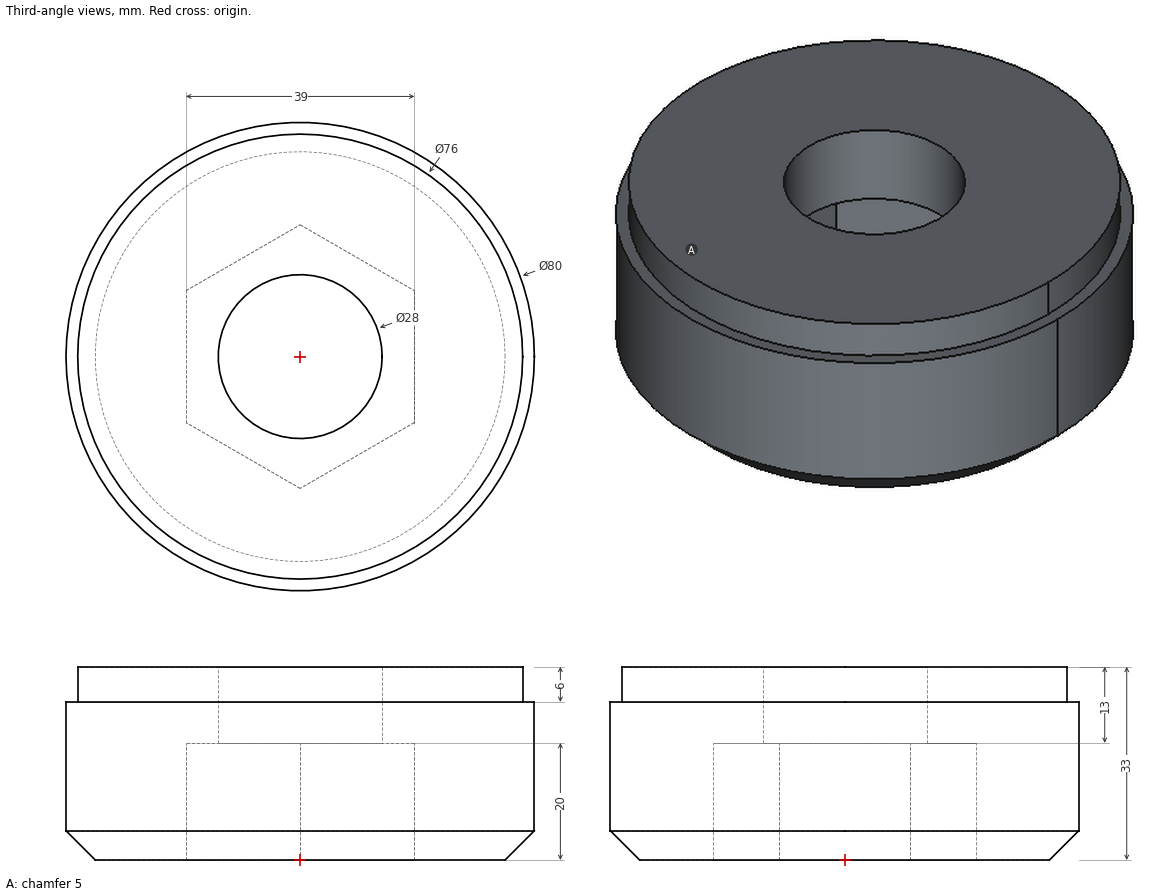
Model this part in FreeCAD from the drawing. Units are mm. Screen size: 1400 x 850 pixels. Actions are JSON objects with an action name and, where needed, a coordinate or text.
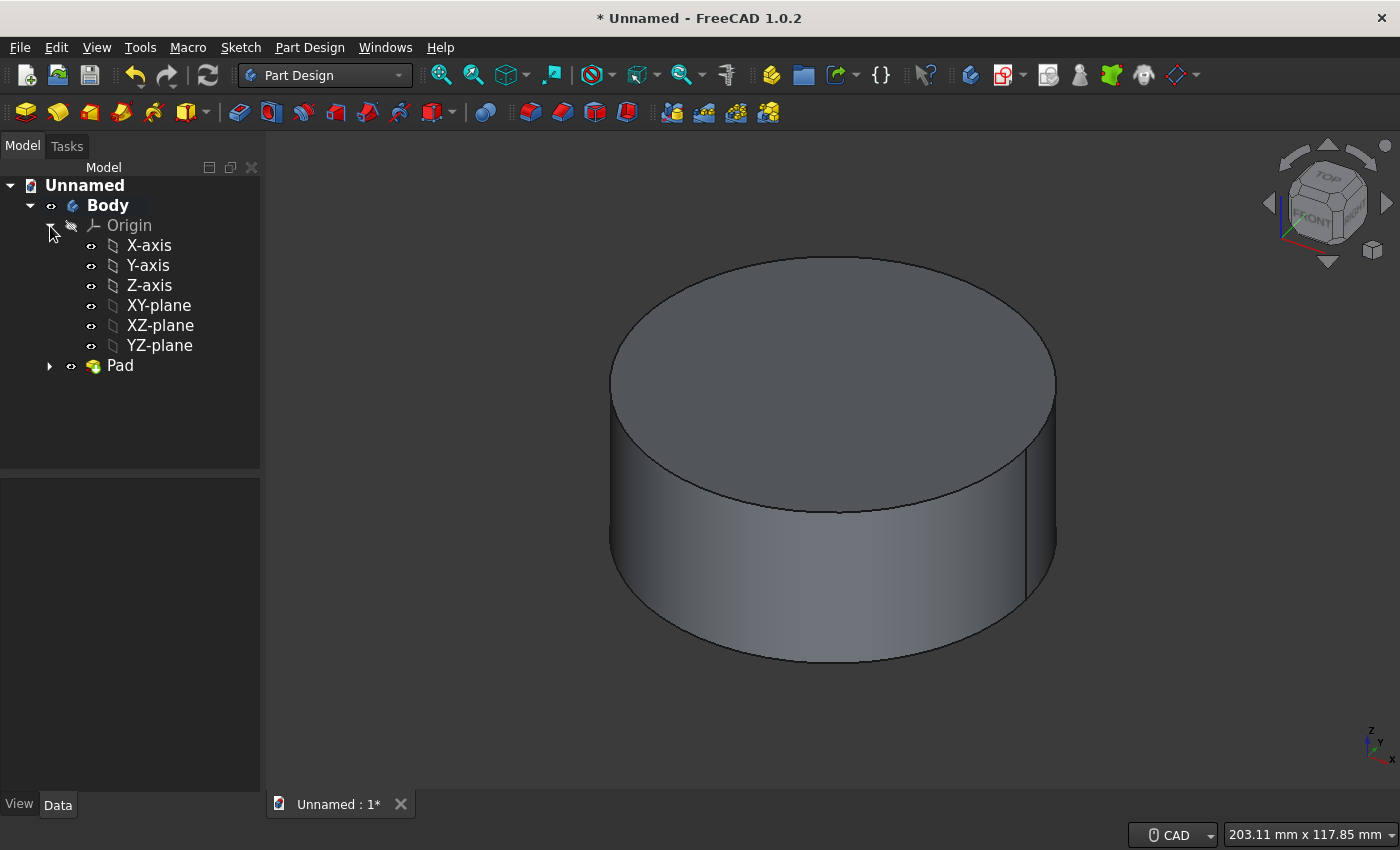
{"action": "left_click", "coordinate": [136, 306]}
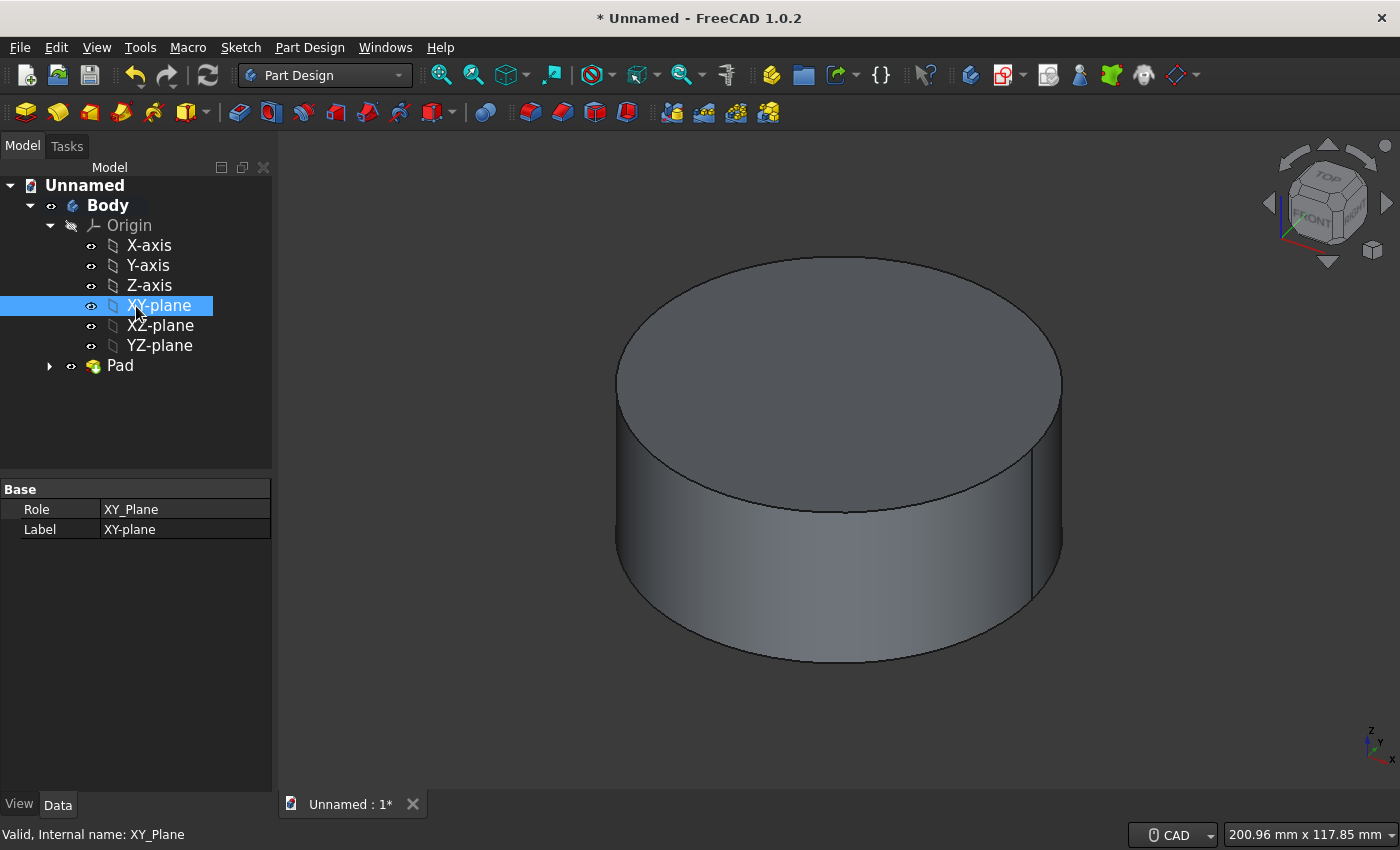
{"action": "left_click", "coordinate": [1176, 76]}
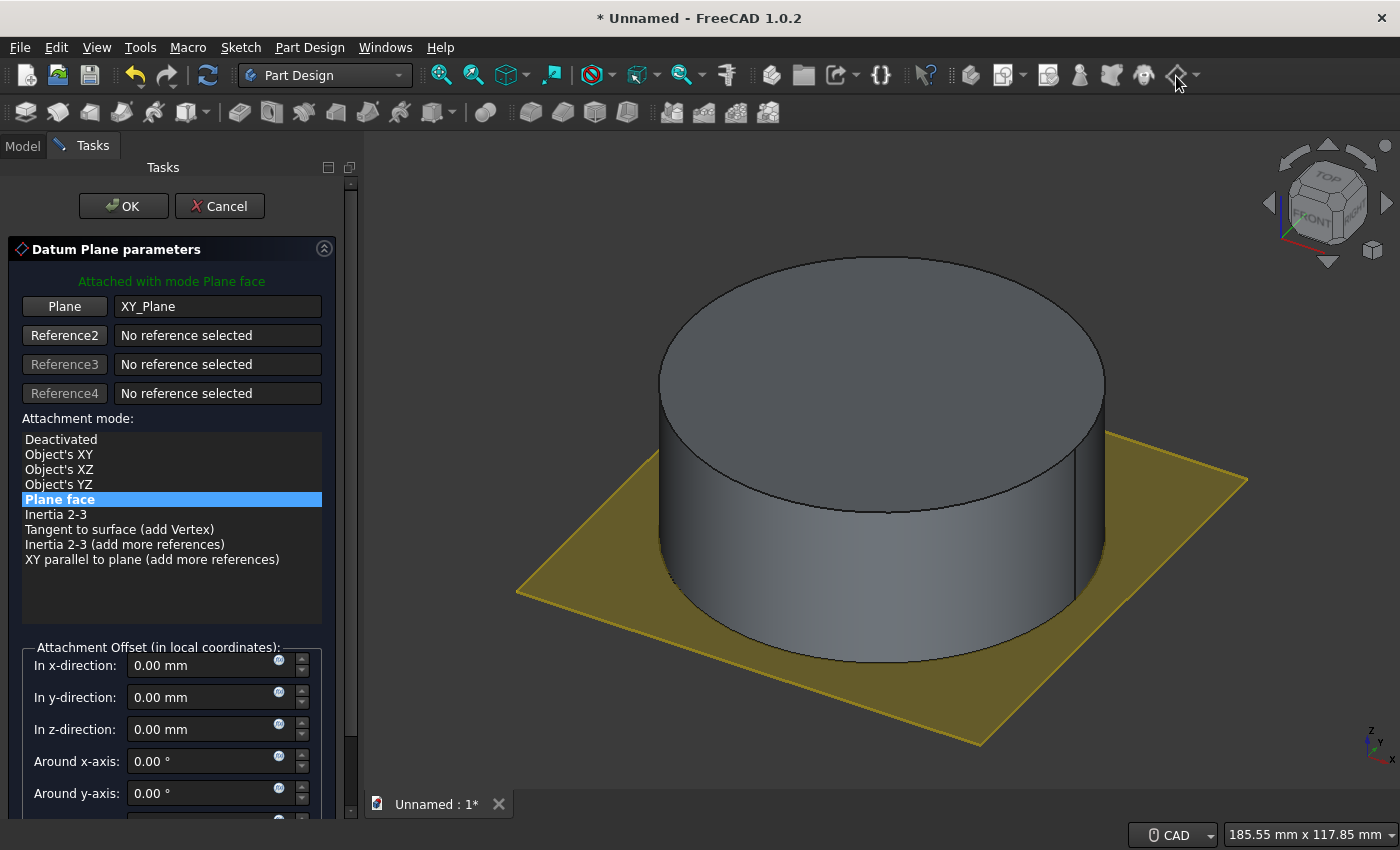
{"action": "triple_click", "coordinate": [210, 729]}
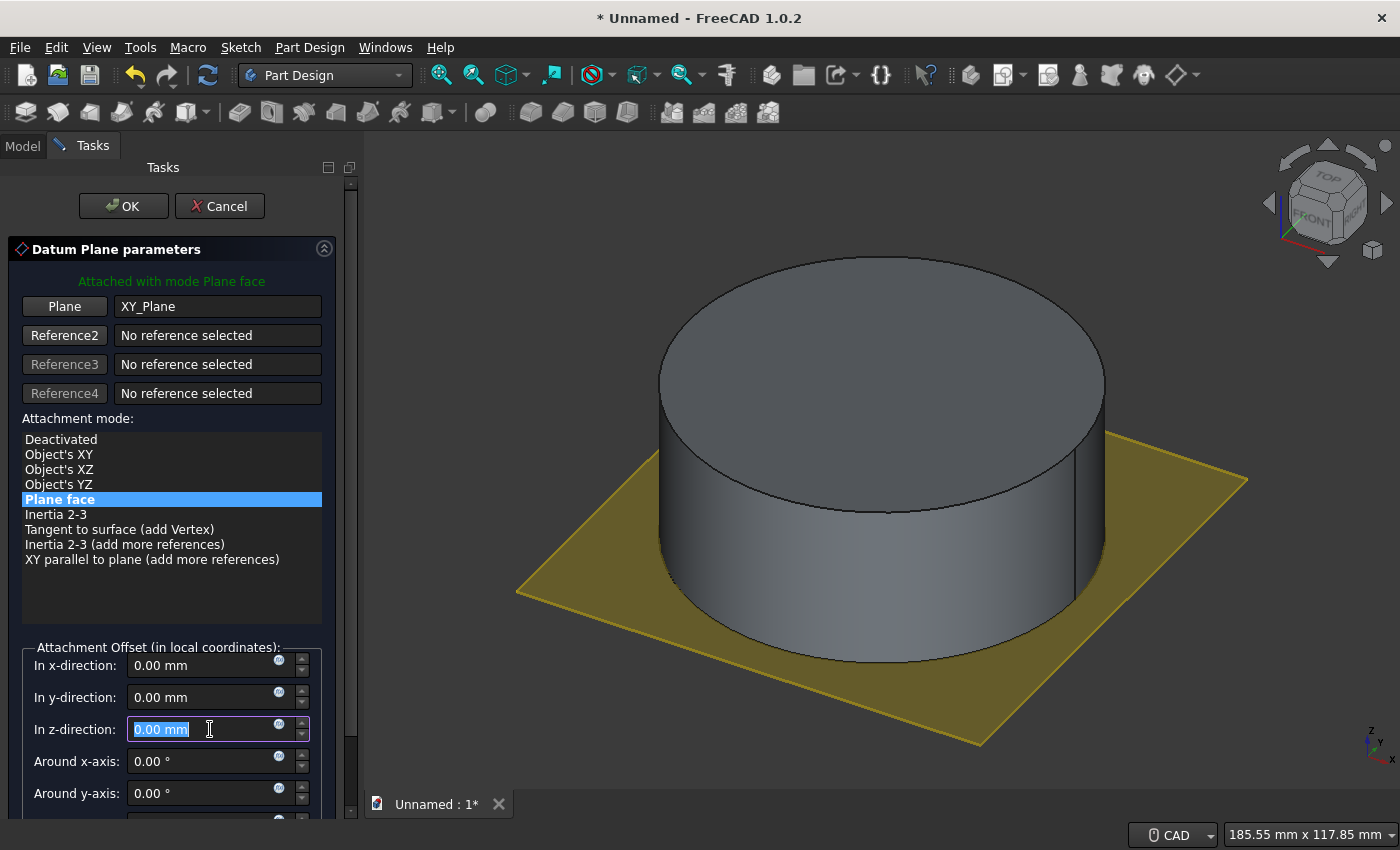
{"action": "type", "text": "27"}
{"action": "key", "text": "Tab"}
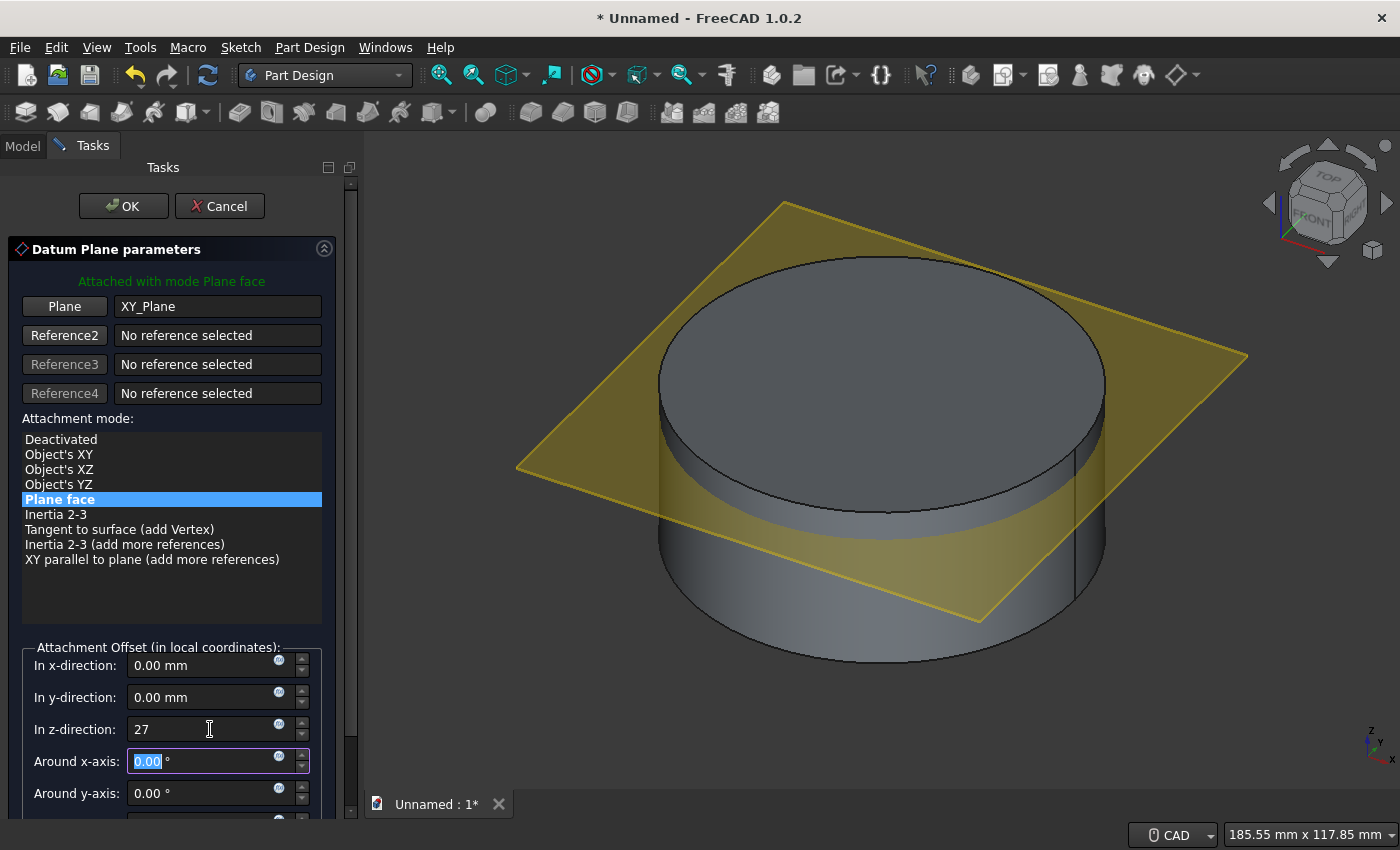
{"action": "left_click", "coordinate": [124, 206]}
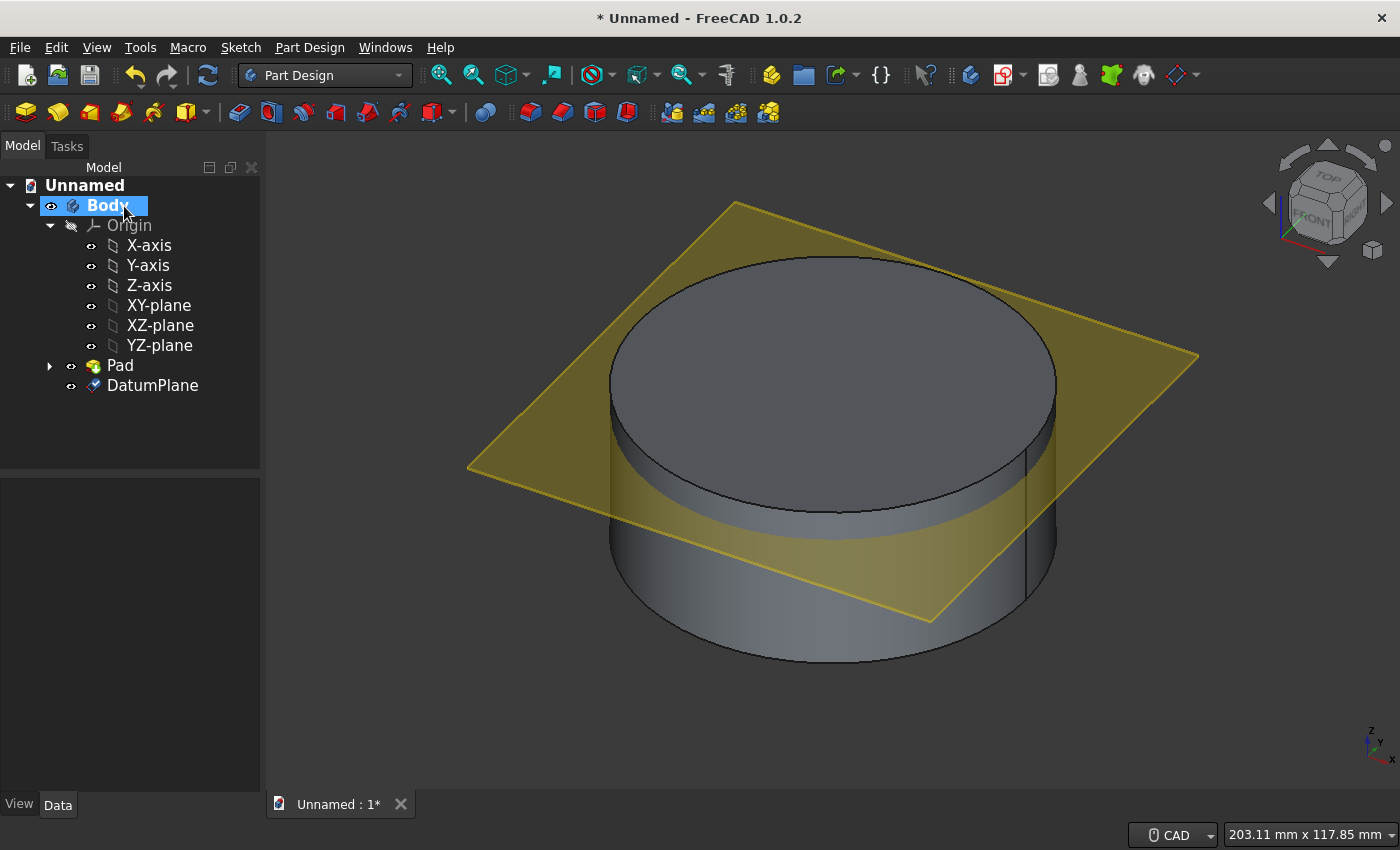
{"action": "left_click", "coordinate": [116, 386]}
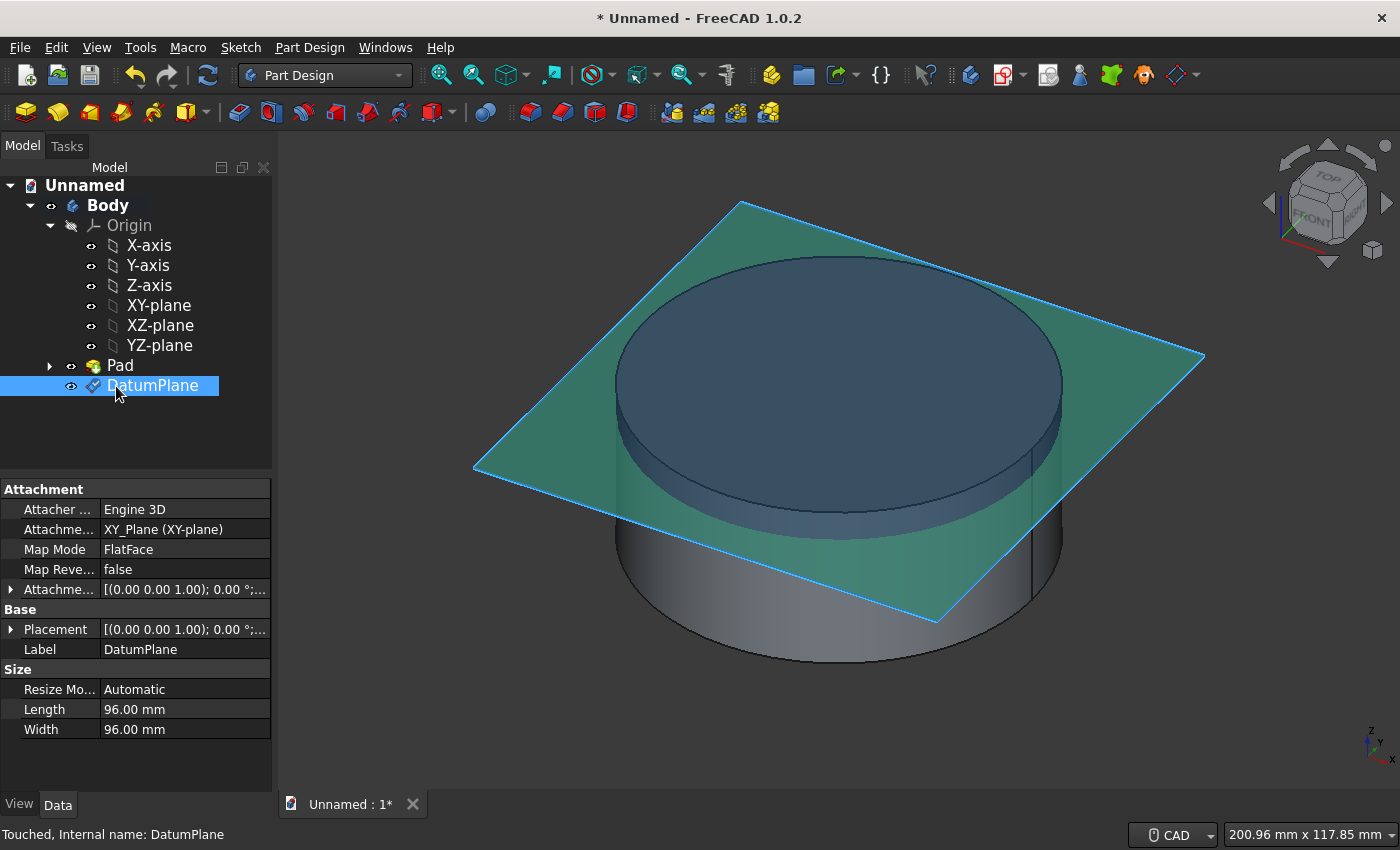
{"action": "left_click", "coordinate": [1004, 76]}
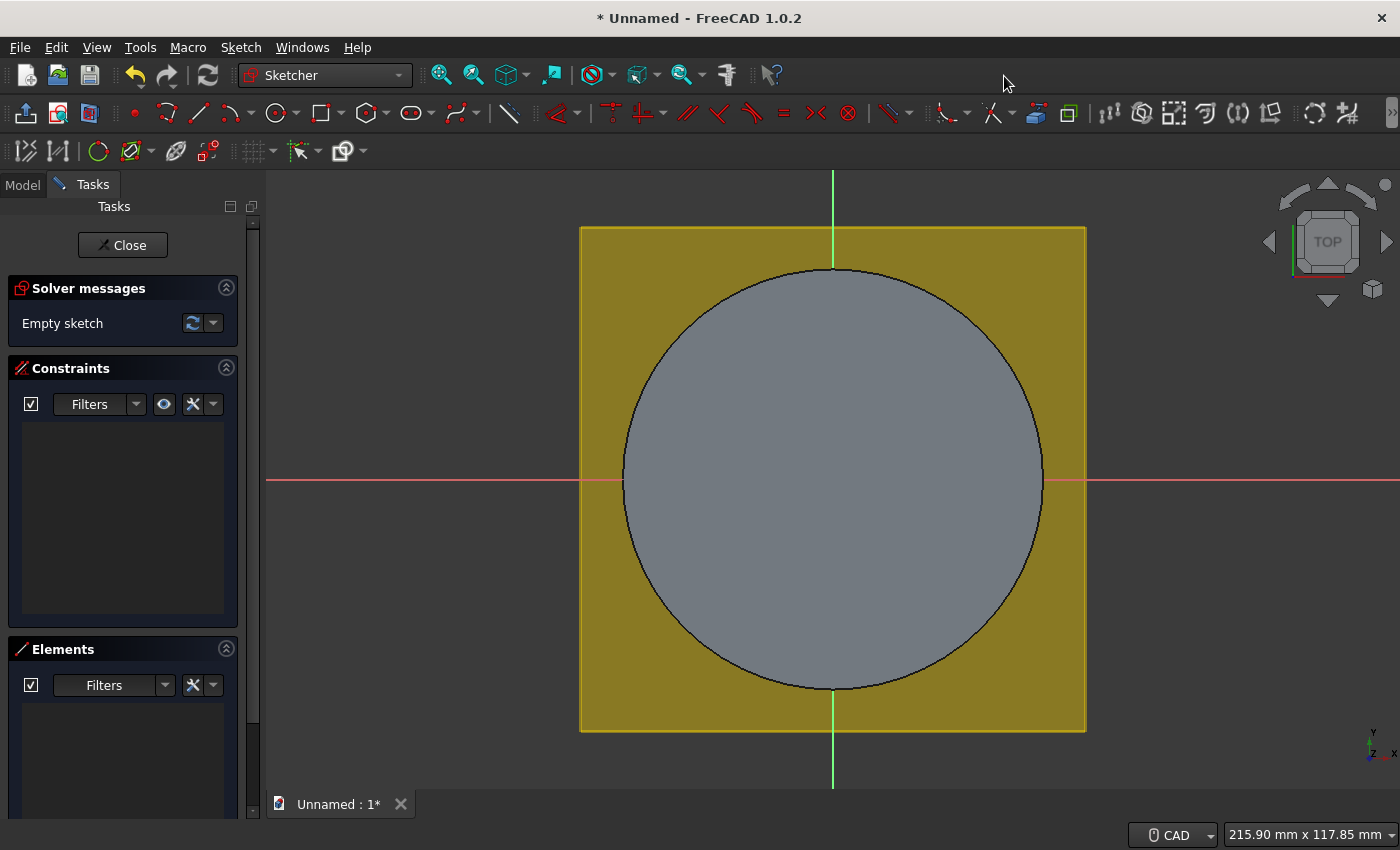
{"action": "left_click", "coordinate": [90, 114]}